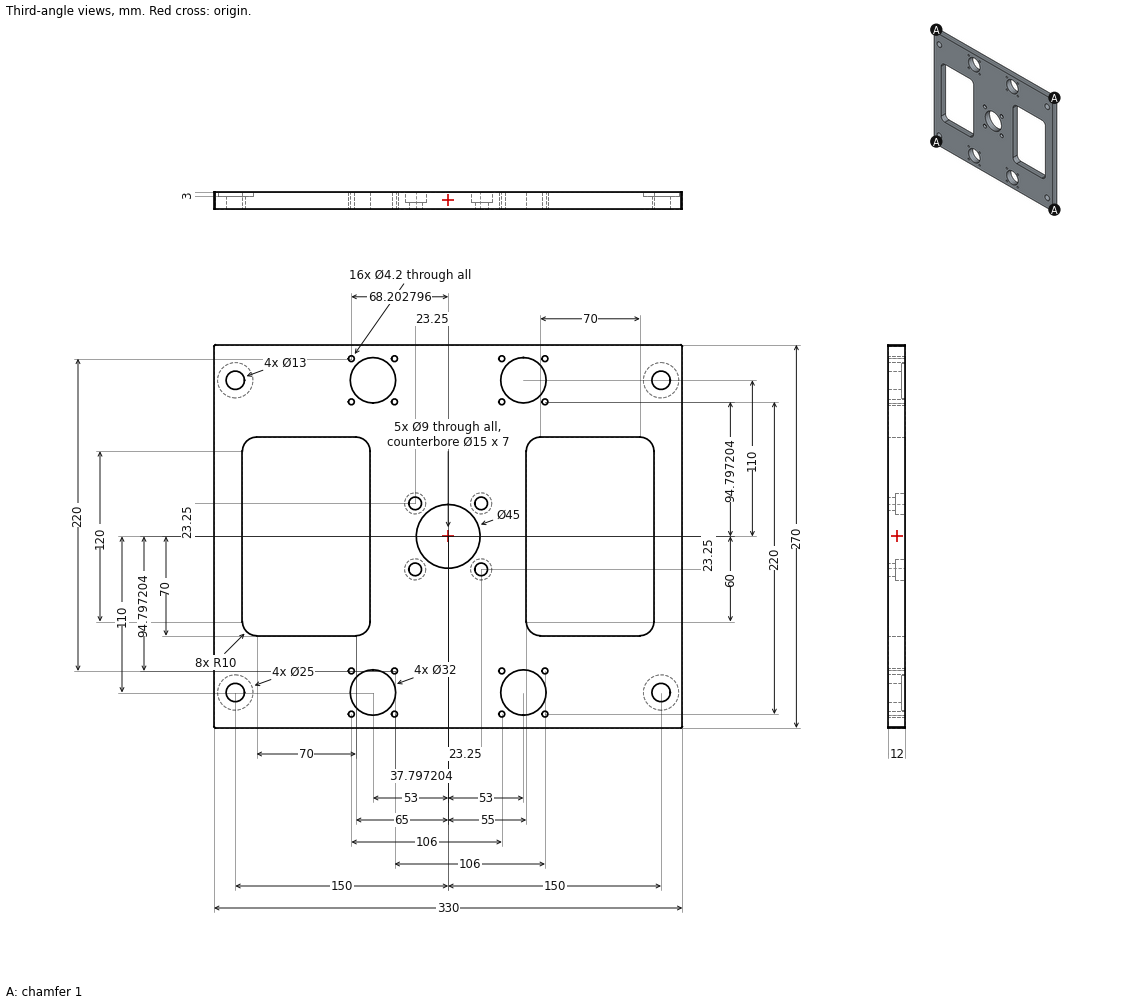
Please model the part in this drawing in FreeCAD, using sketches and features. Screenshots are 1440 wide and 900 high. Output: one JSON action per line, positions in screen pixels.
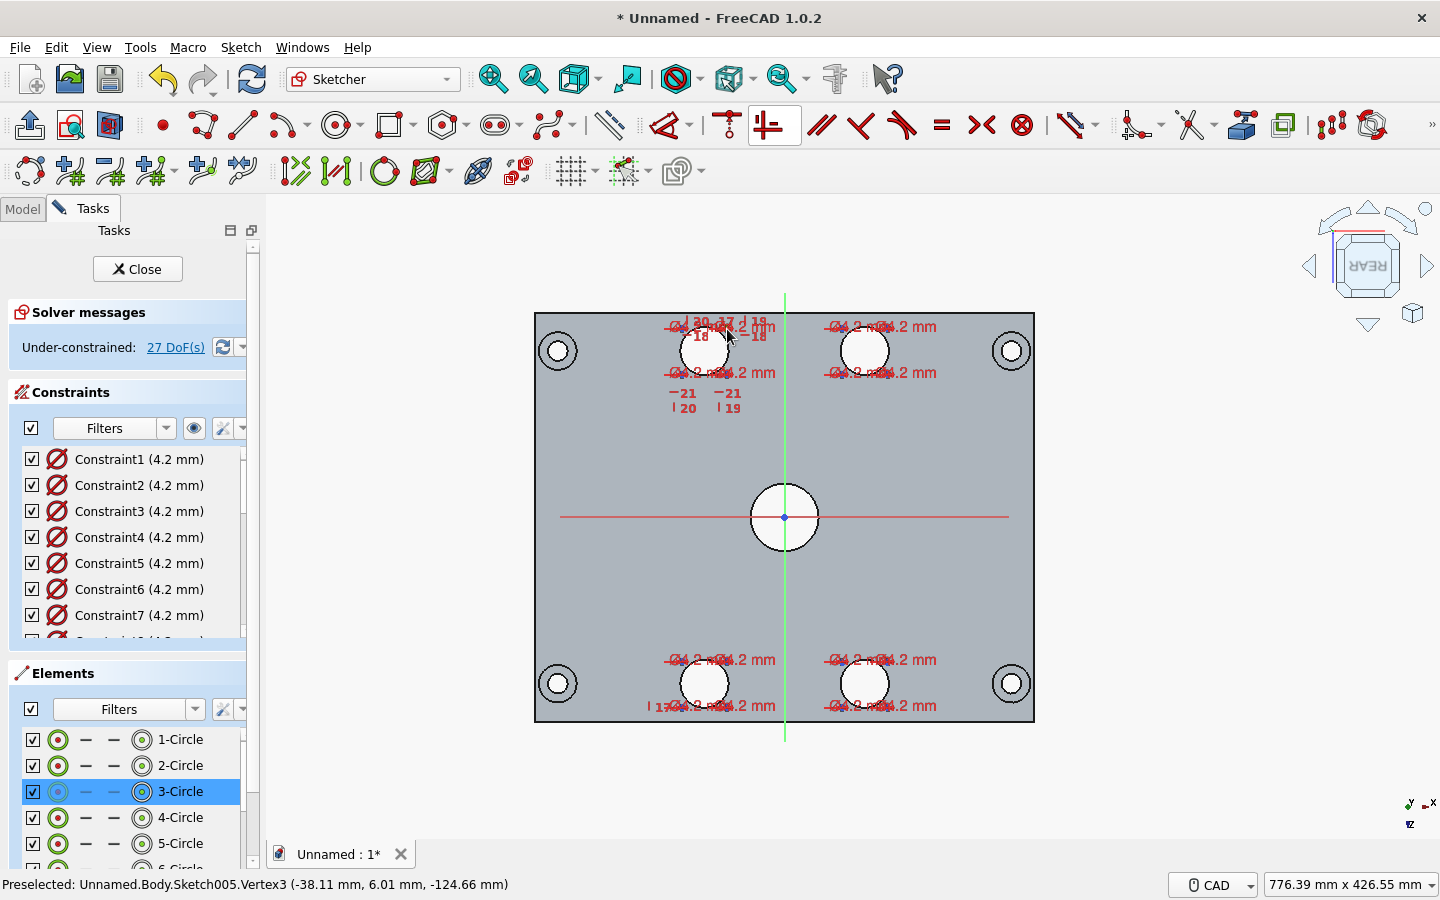
{"action": "left_click", "coordinate": [842, 329]}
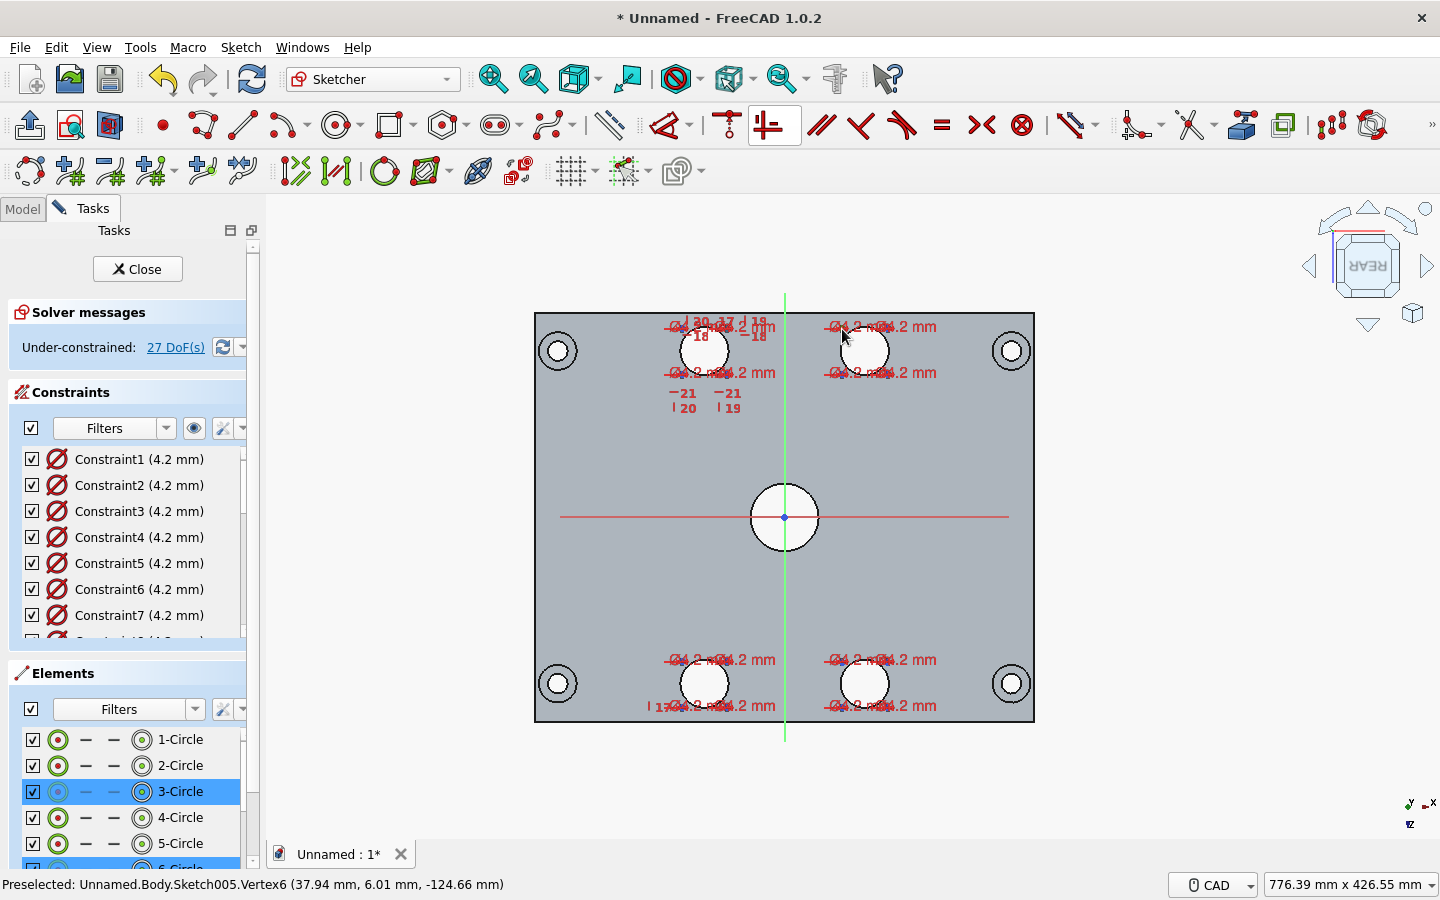
{"action": "left_click", "coordinate": [796, 126]}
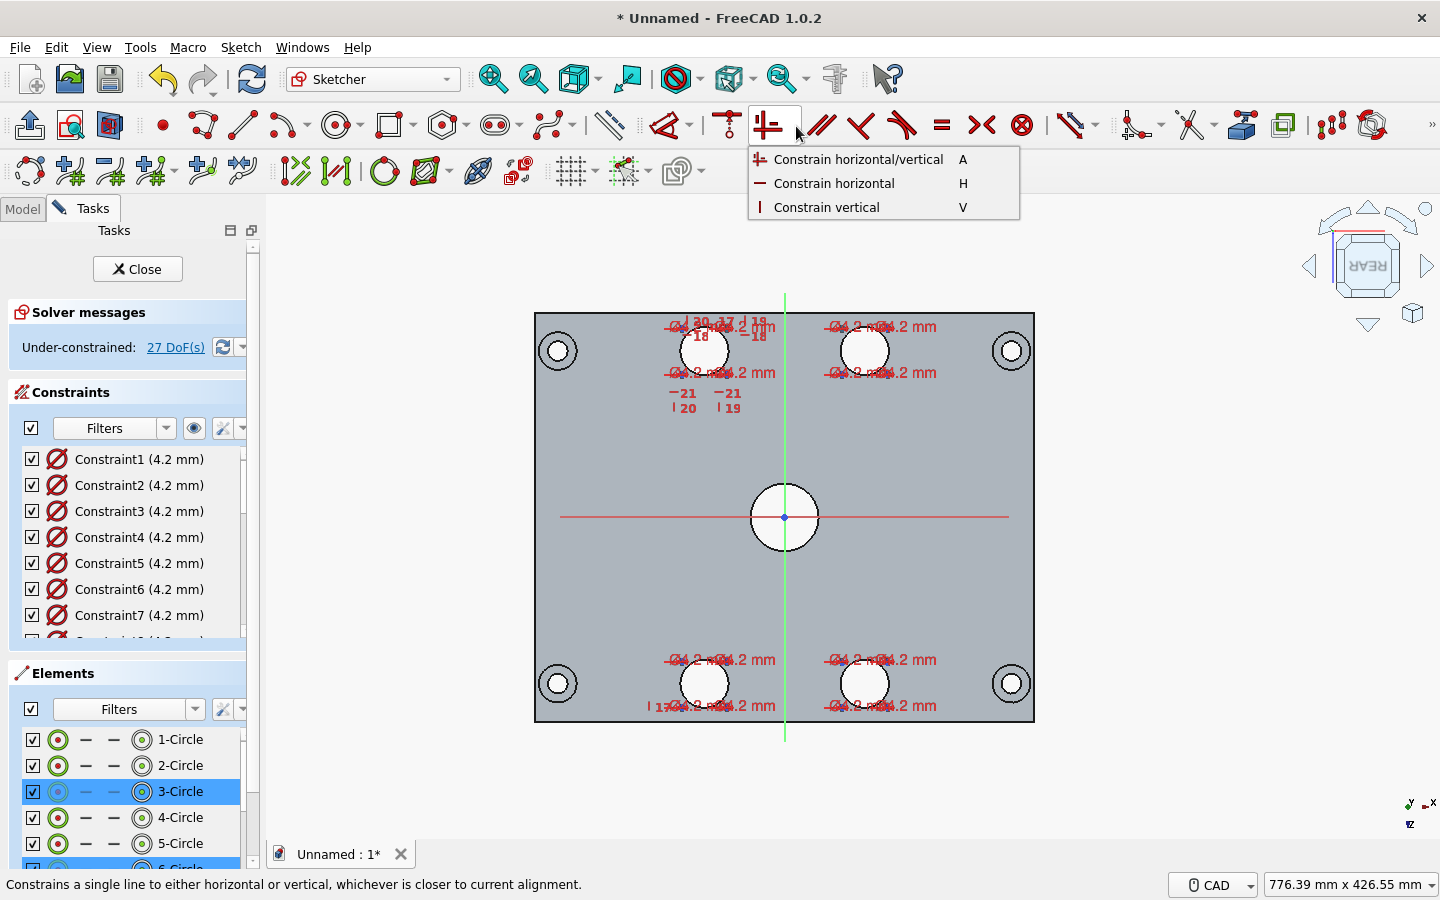
{"action": "left_click", "coordinate": [884, 183]}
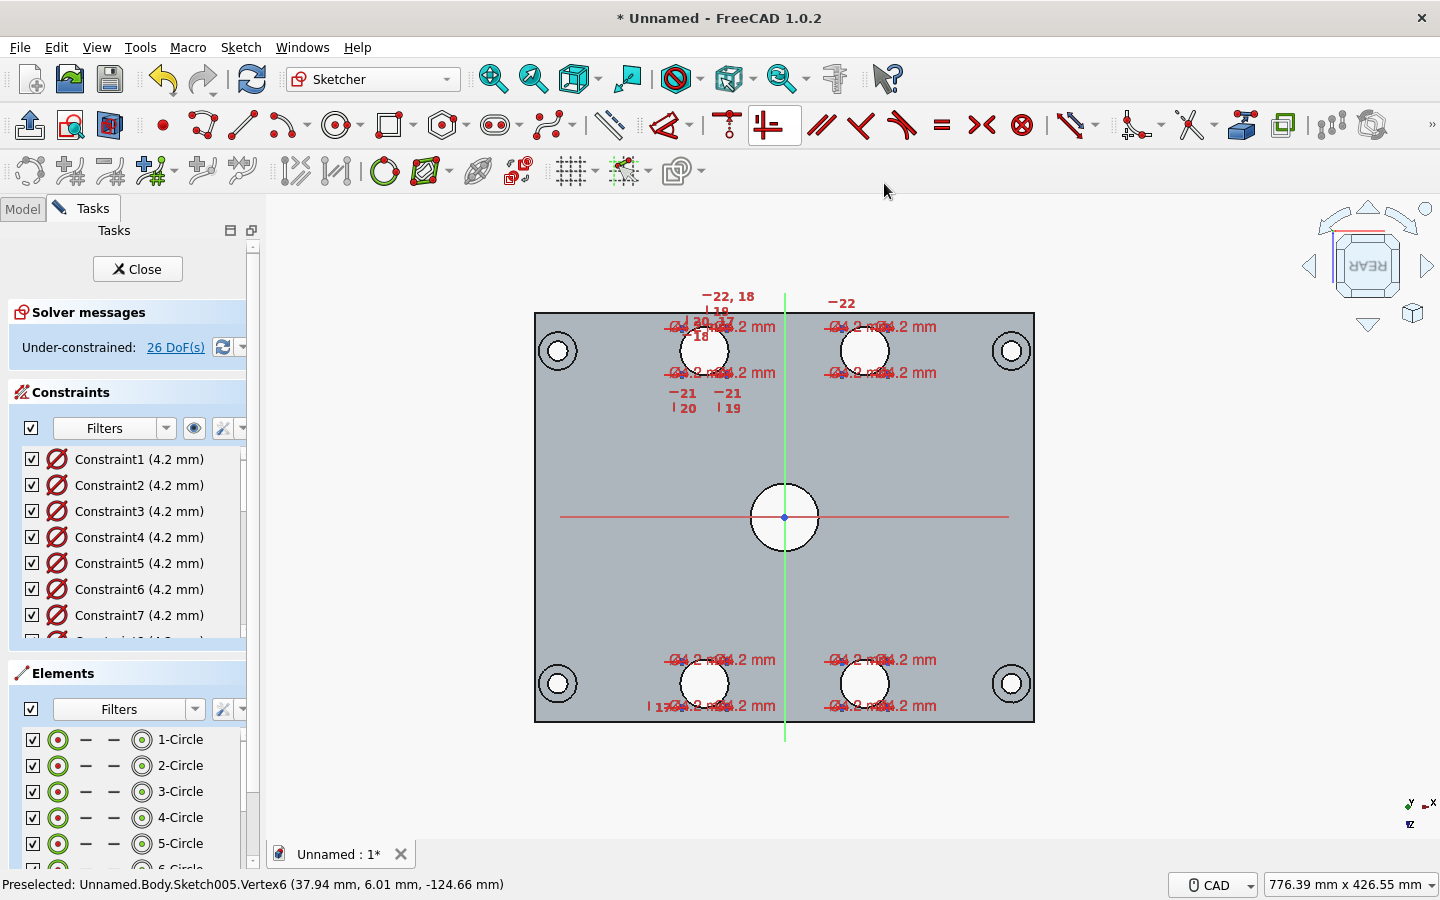
{"action": "left_click", "coordinate": [842, 329]}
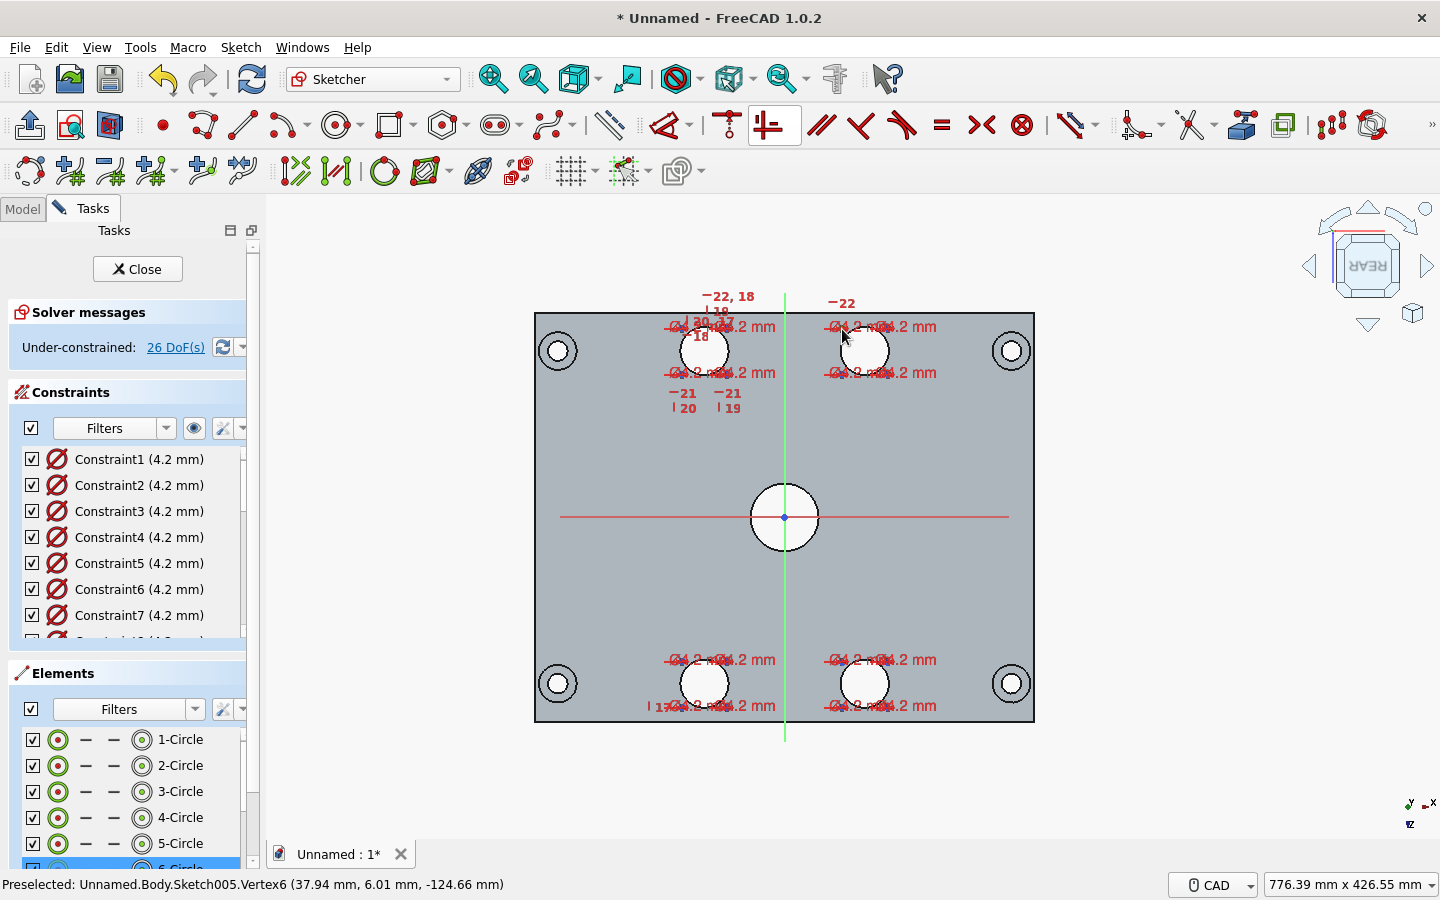
{"action": "left_click", "coordinate": [842, 375]}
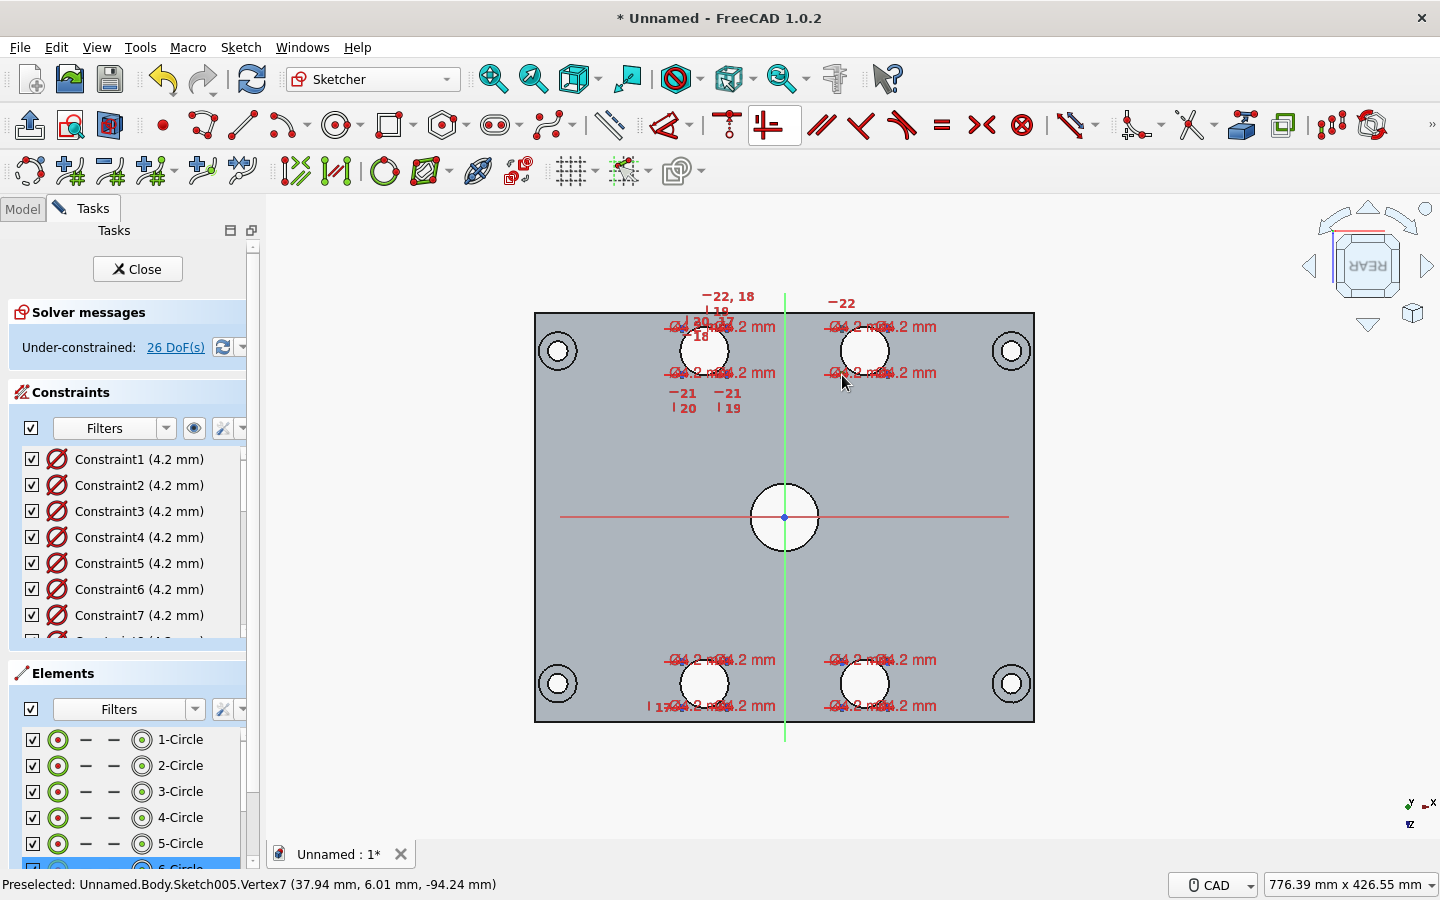
{"action": "left_click", "coordinate": [796, 126]}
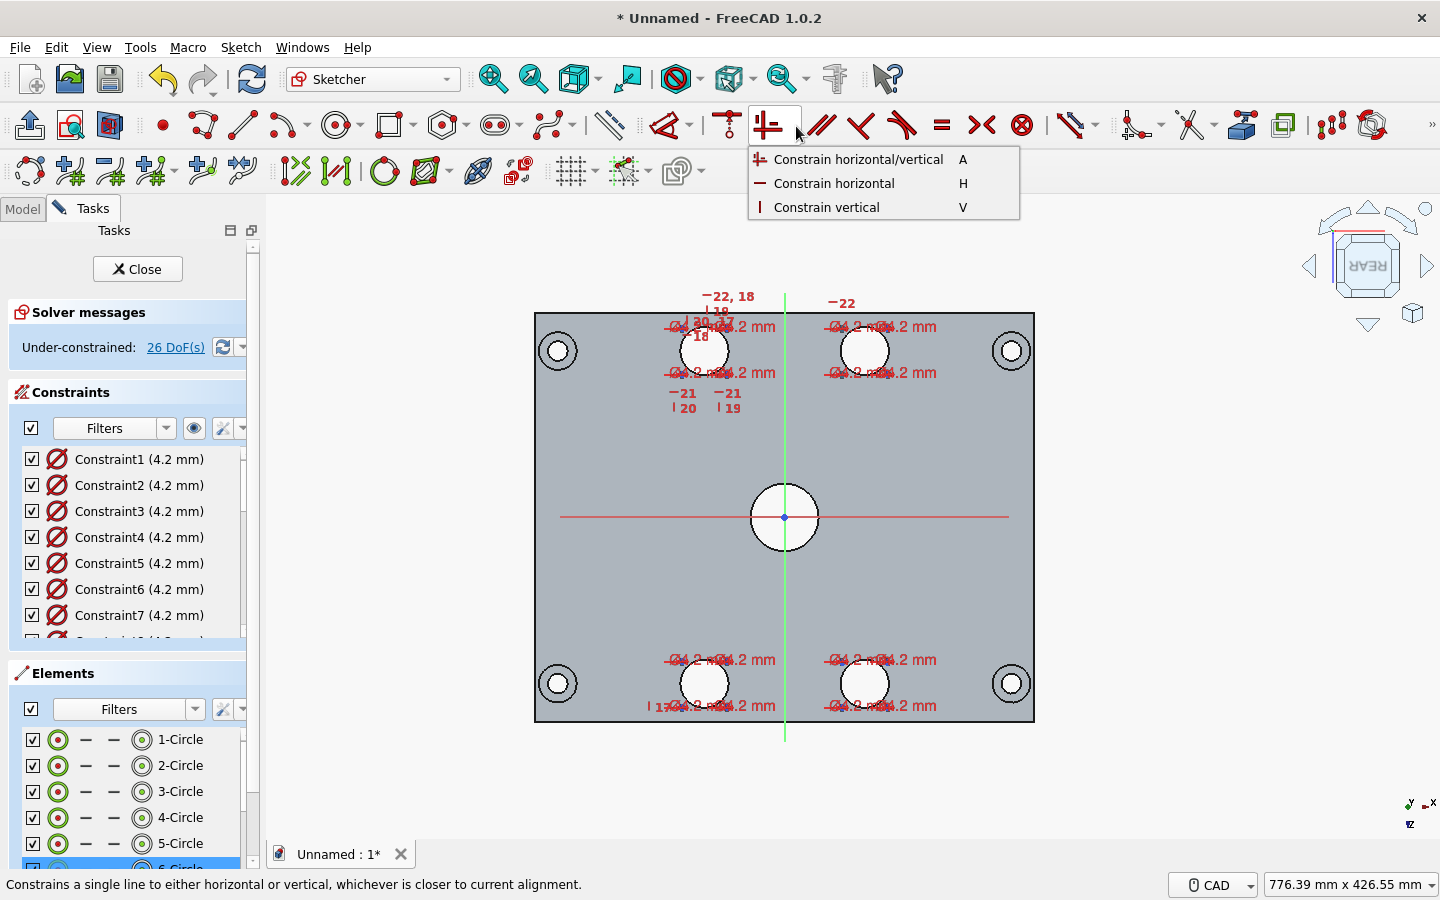
{"action": "left_click", "coordinate": [884, 207]}